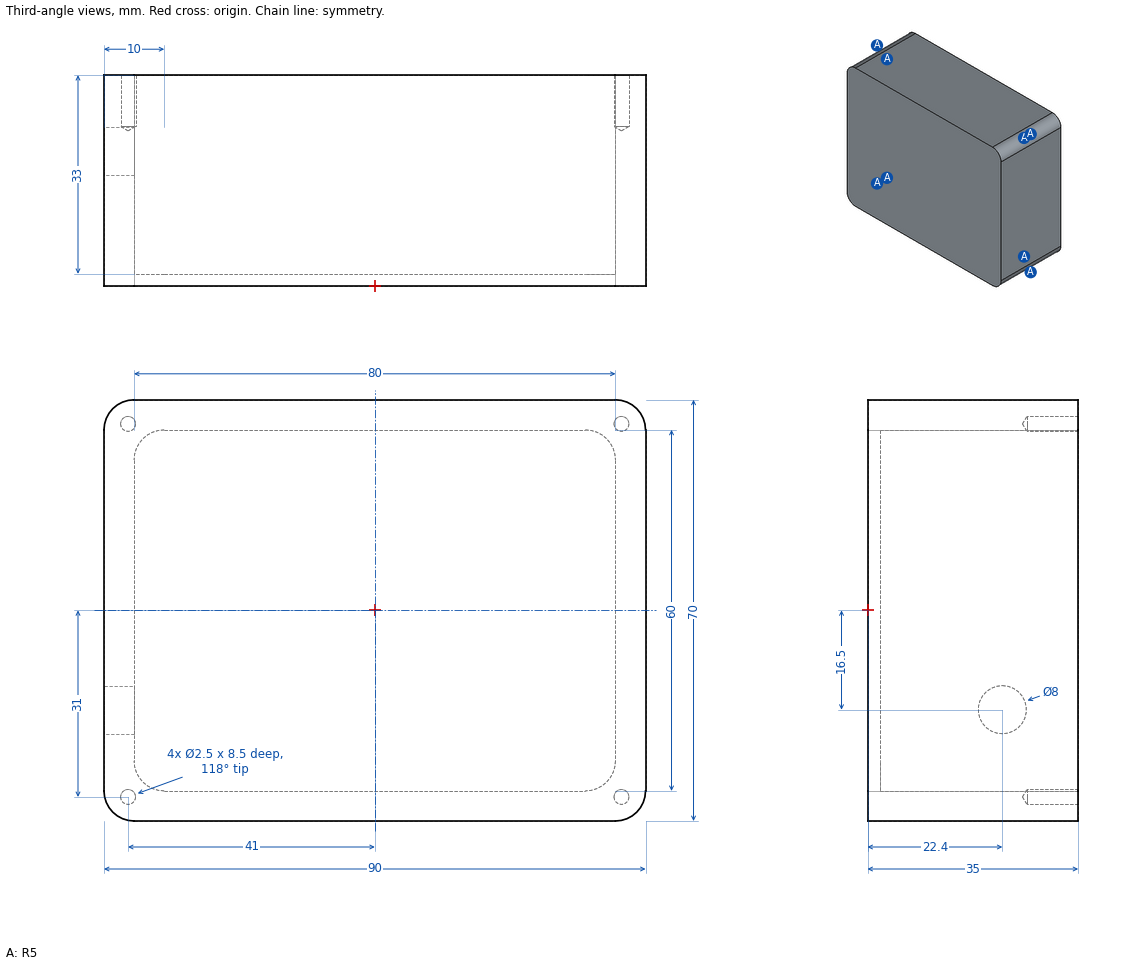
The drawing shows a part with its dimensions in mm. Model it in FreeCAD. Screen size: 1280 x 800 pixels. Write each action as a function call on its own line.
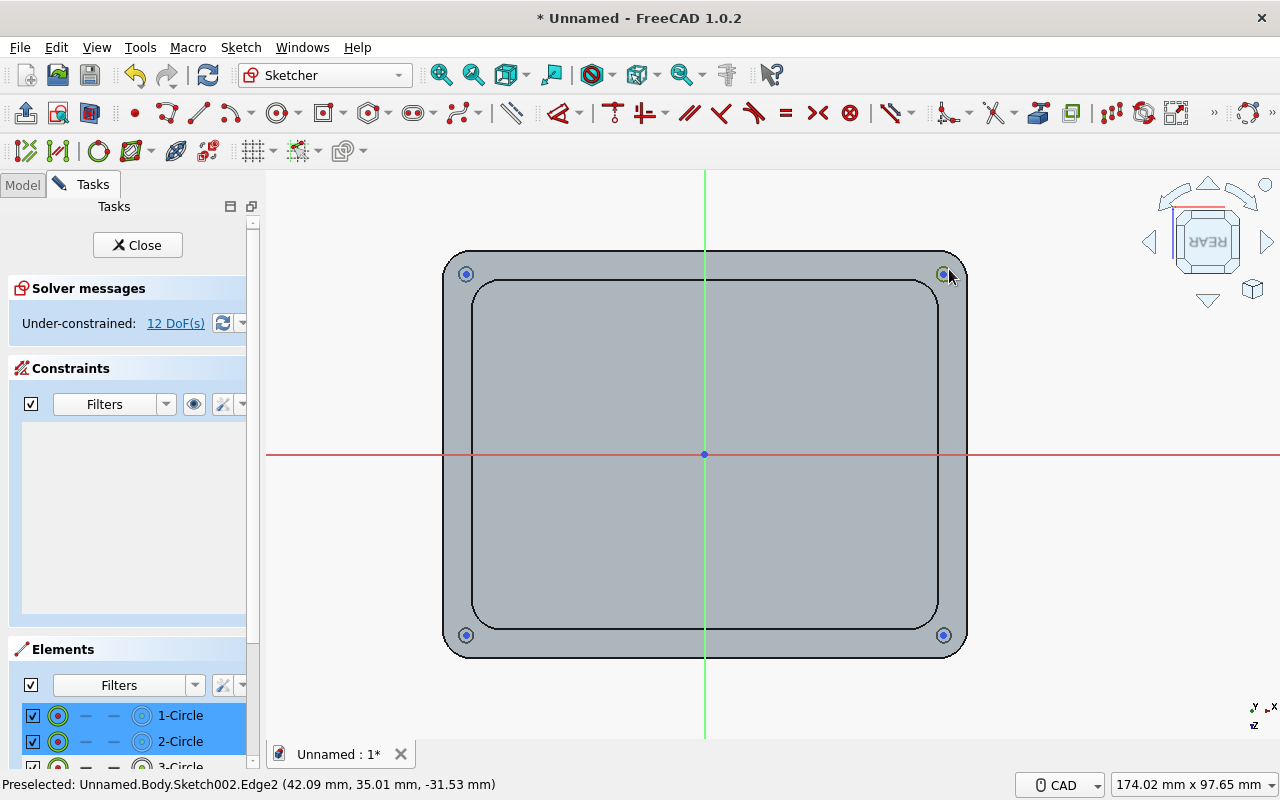
scroll(949, 630, up, 4)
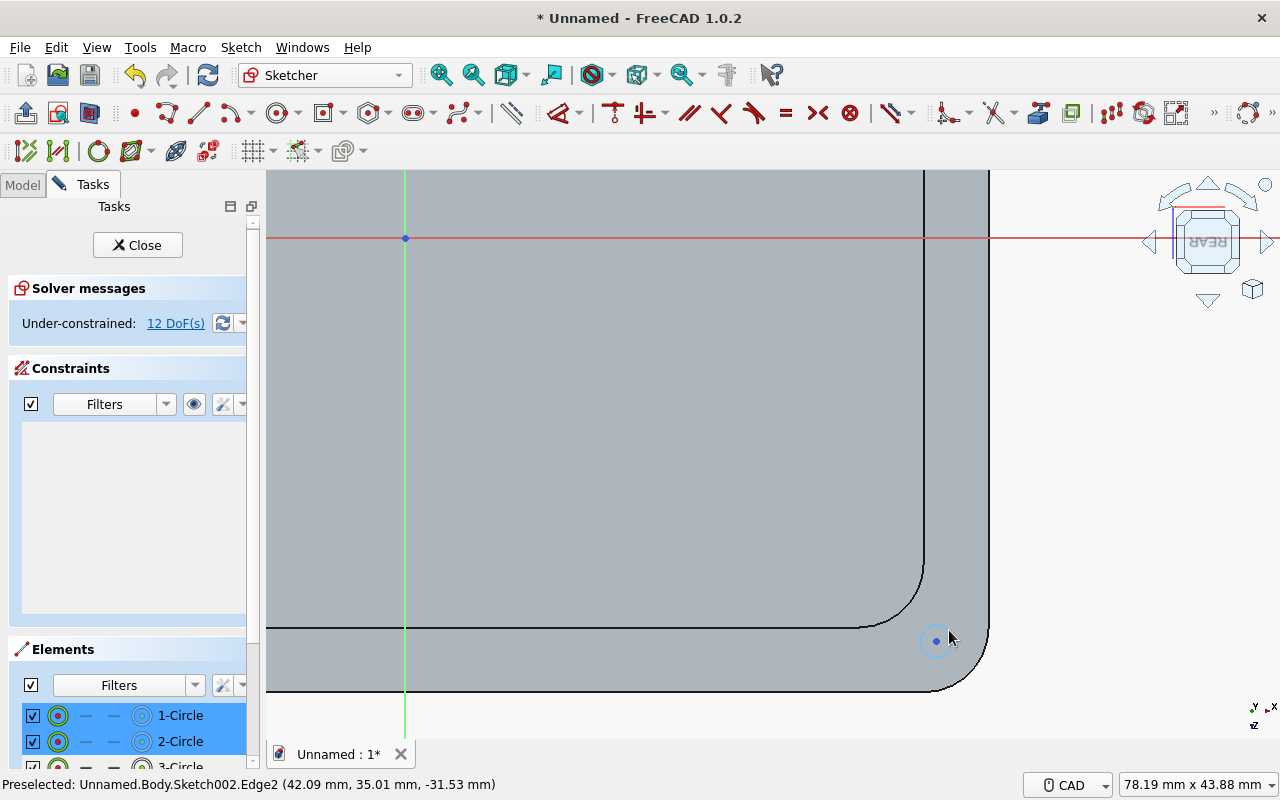
click(948, 630)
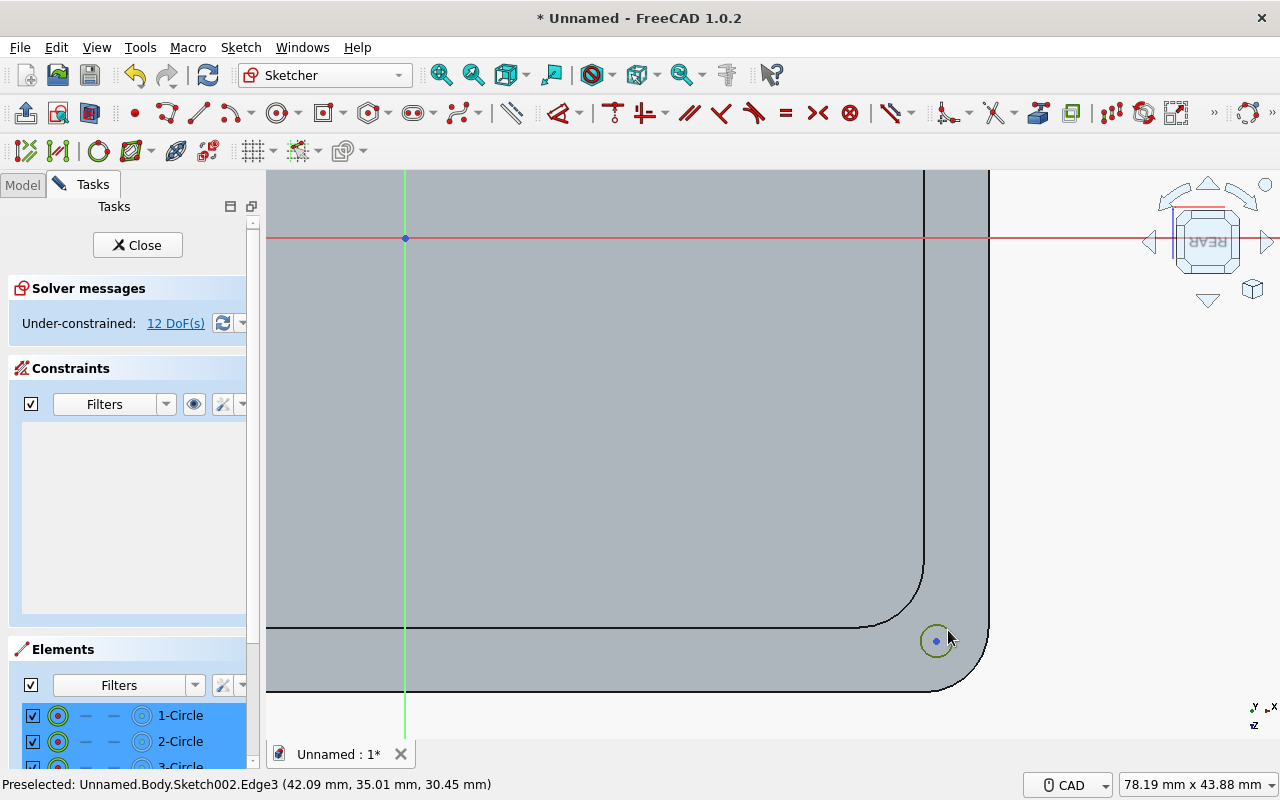
scroll(949, 631, down, 4)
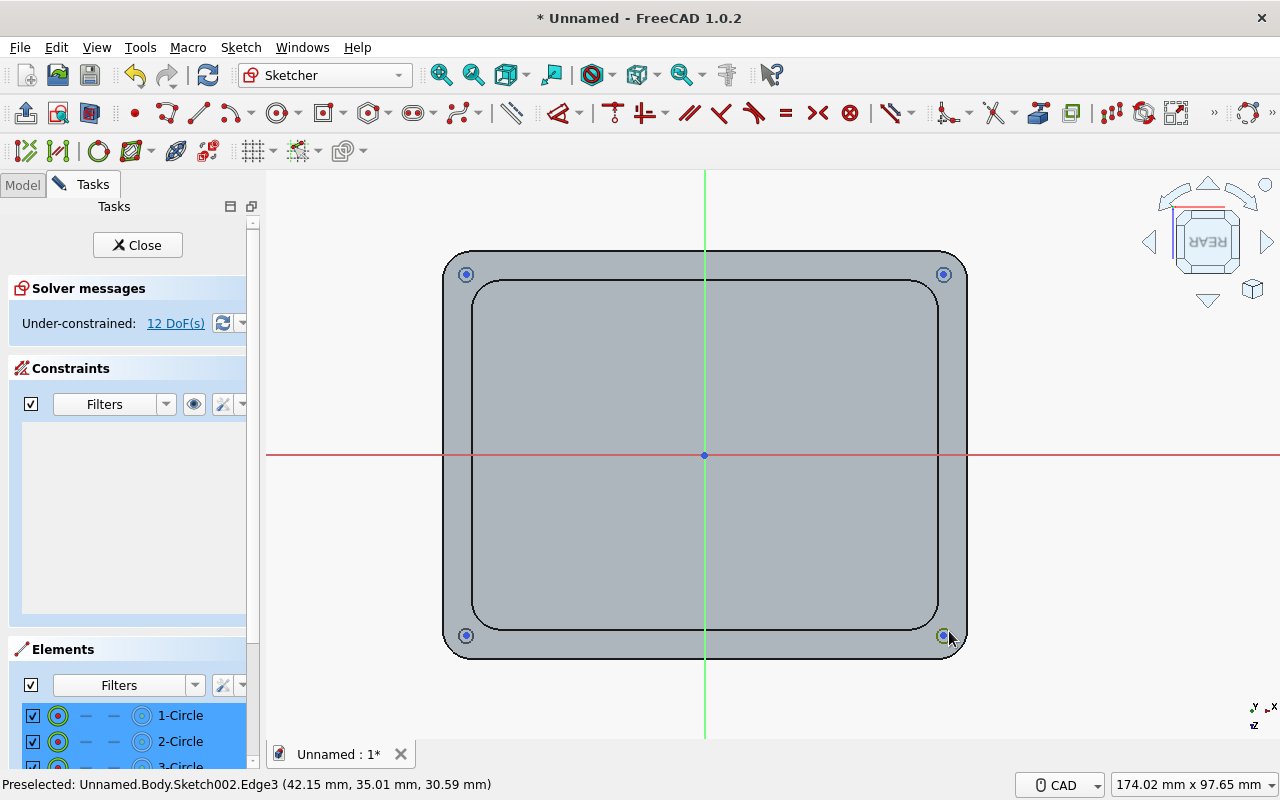
scroll(471, 631, up, 4)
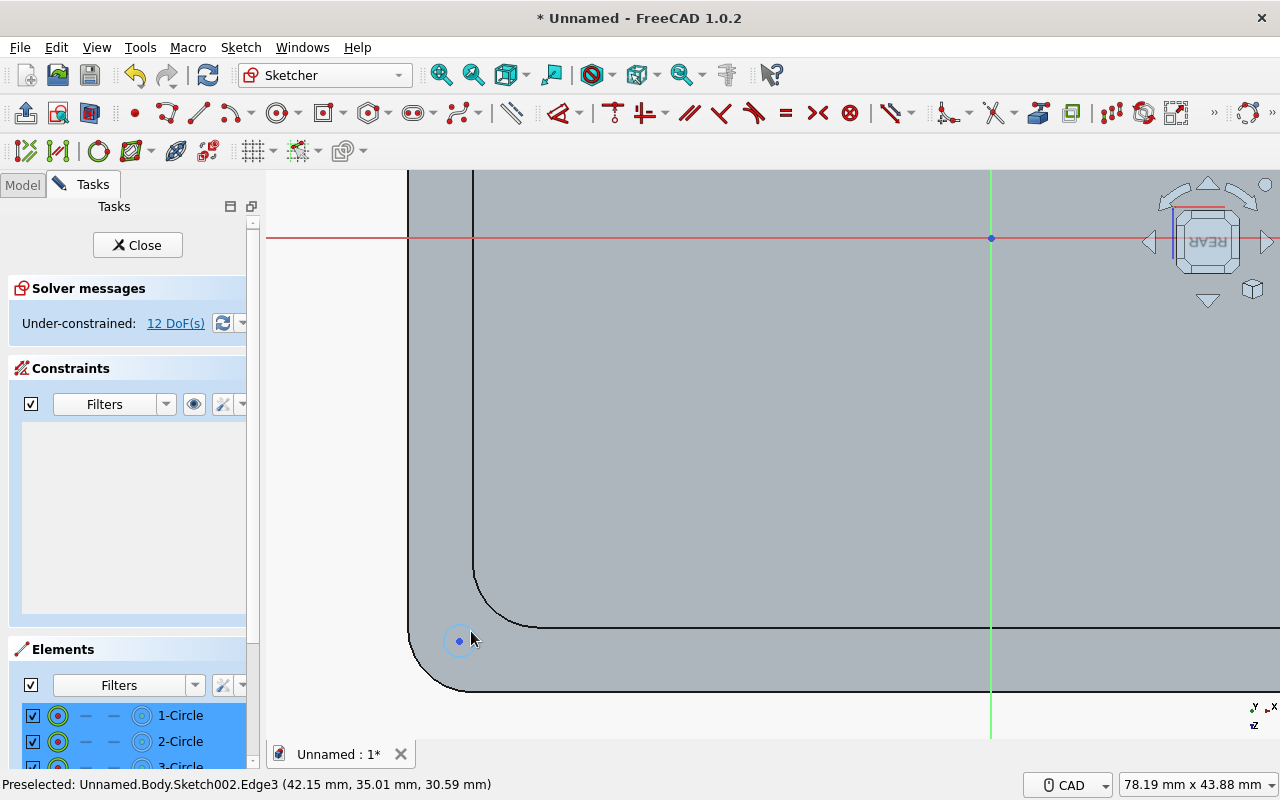
click(471, 630)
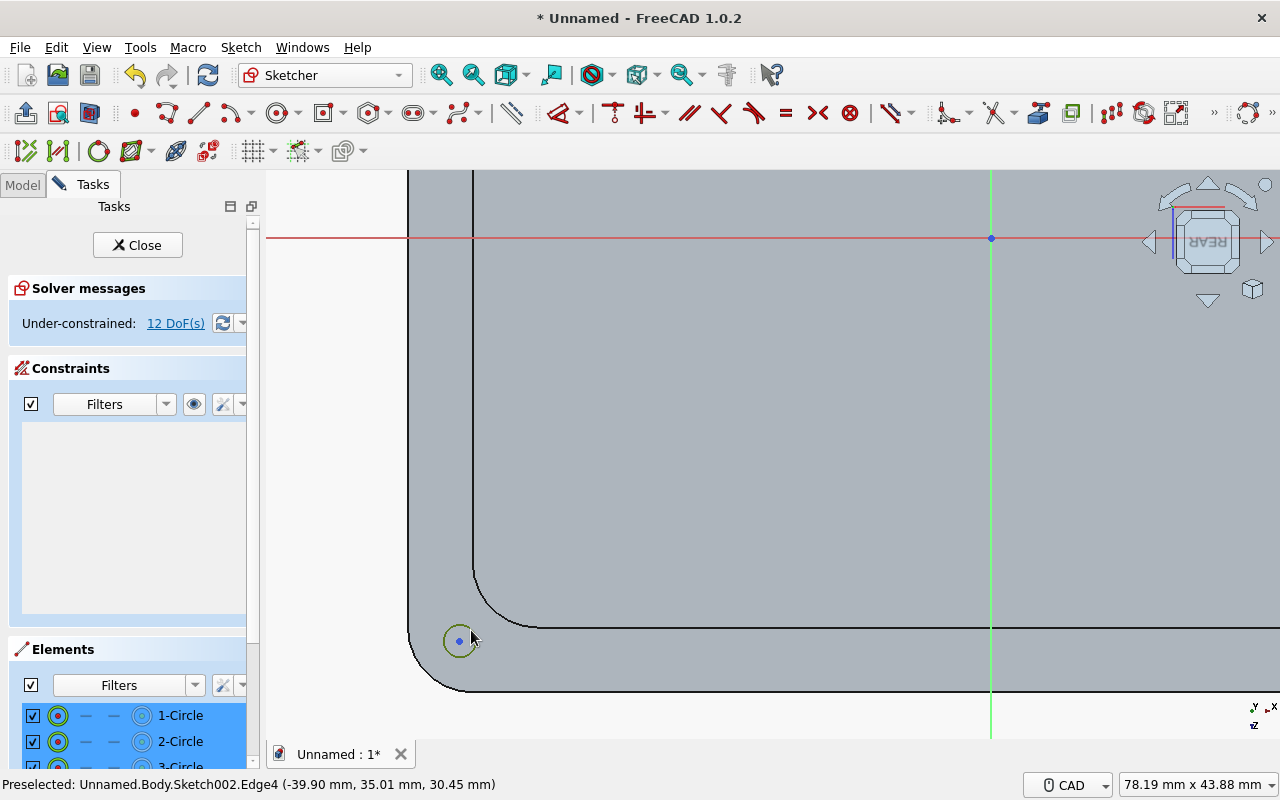
click(786, 114)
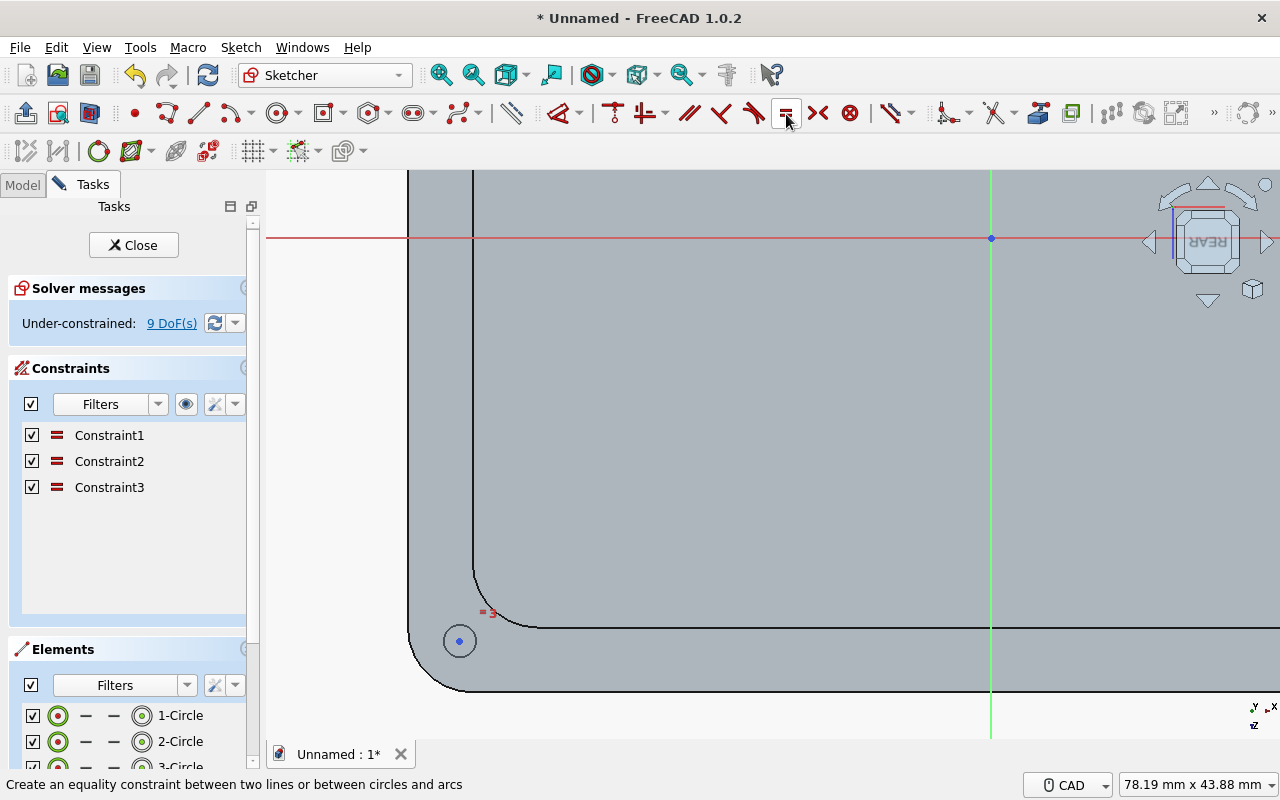
scroll(470, 631, down, 4)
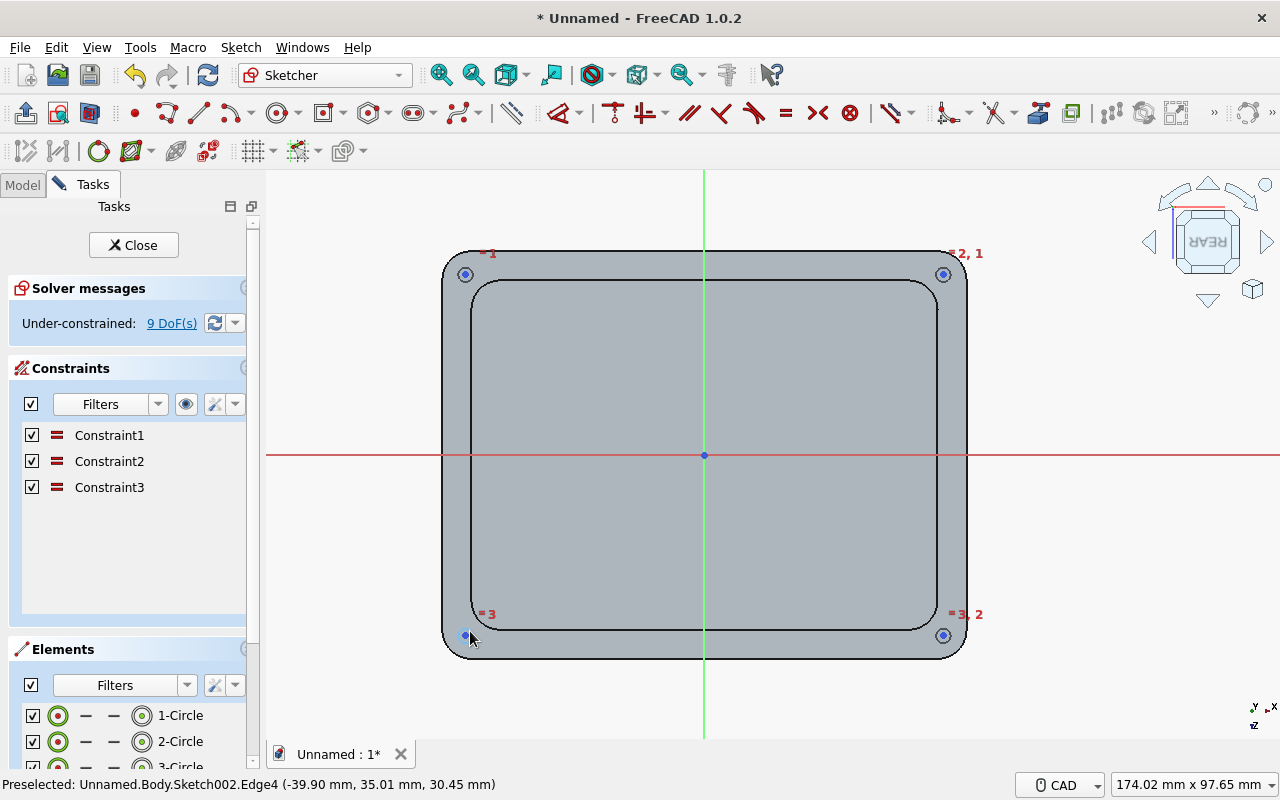
click(466, 275)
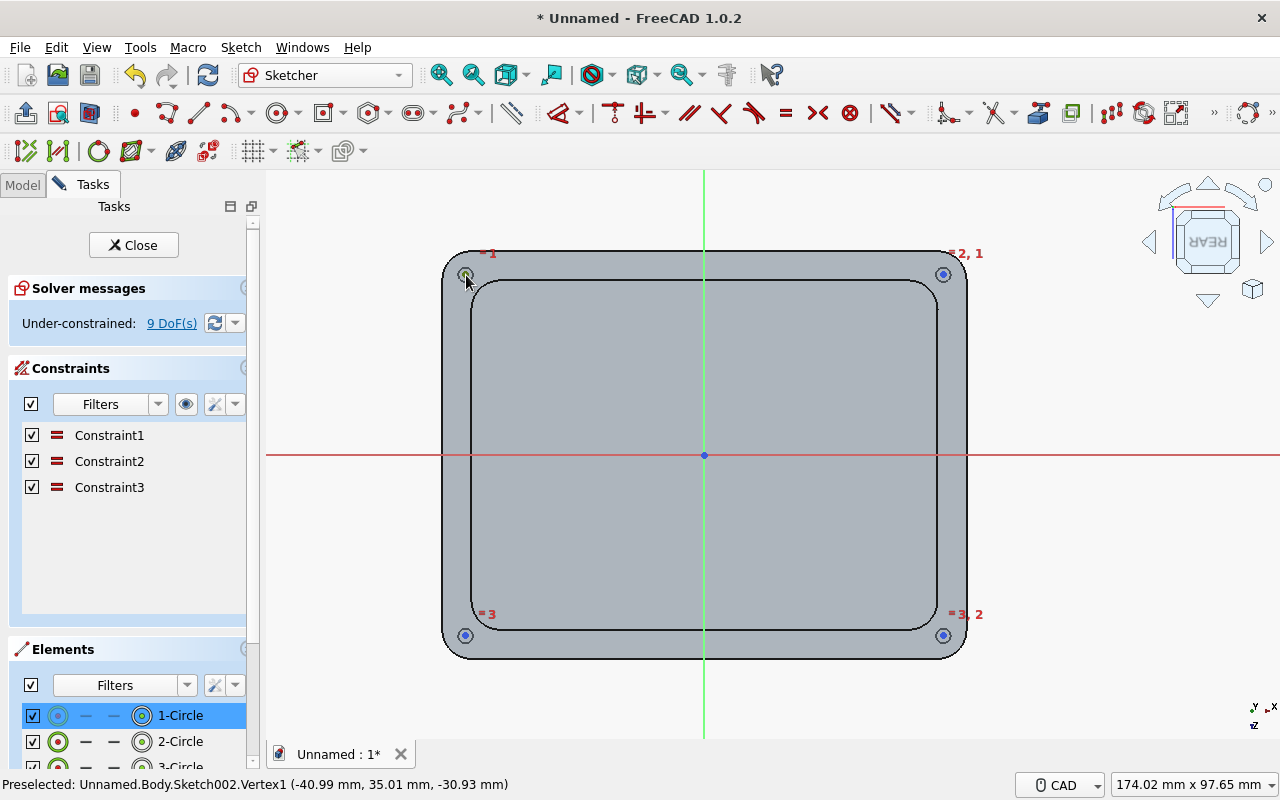
click(943, 275)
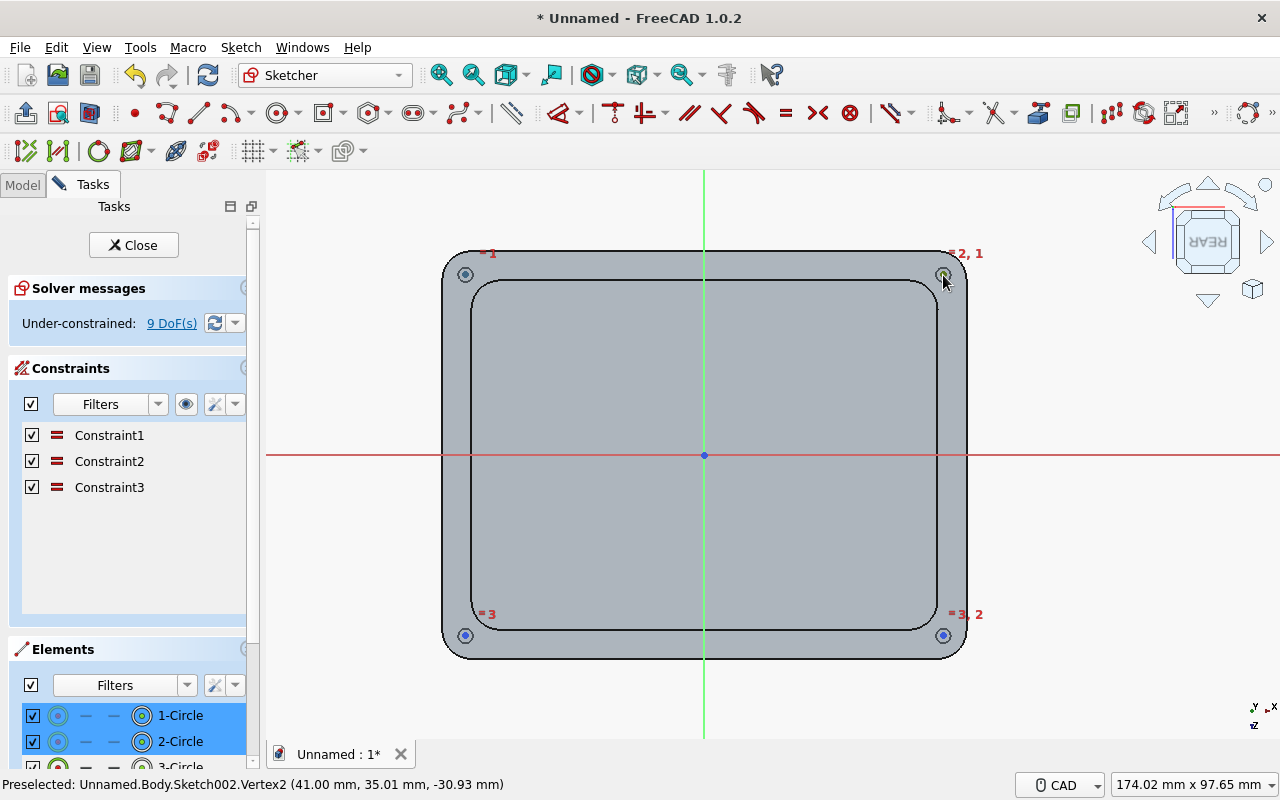
click(704, 674)